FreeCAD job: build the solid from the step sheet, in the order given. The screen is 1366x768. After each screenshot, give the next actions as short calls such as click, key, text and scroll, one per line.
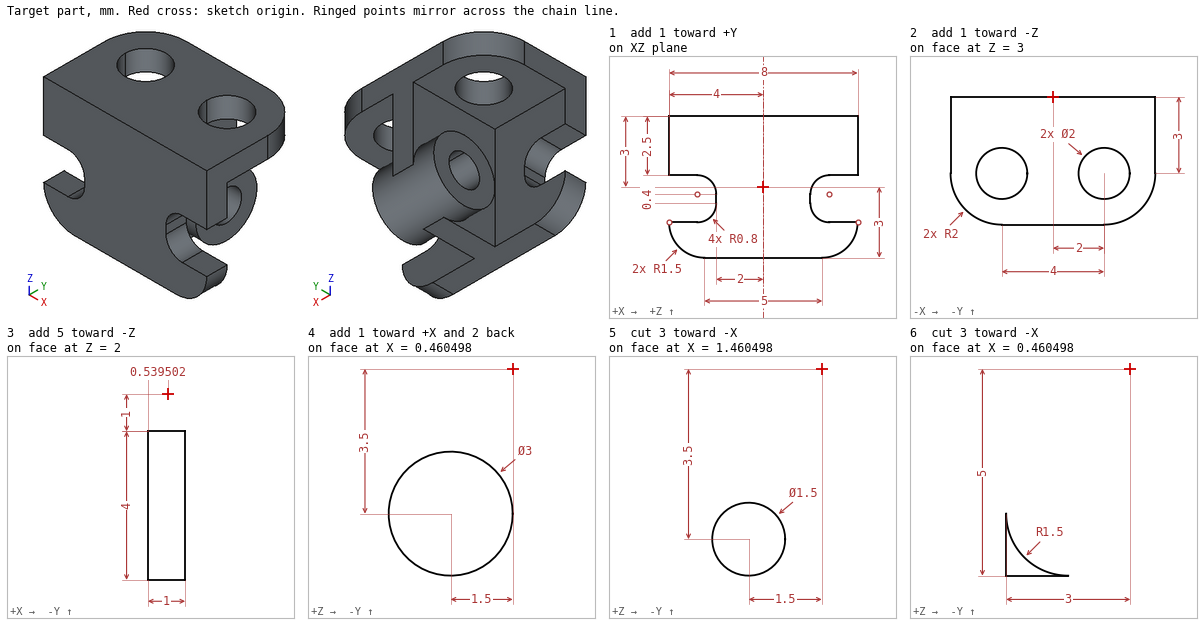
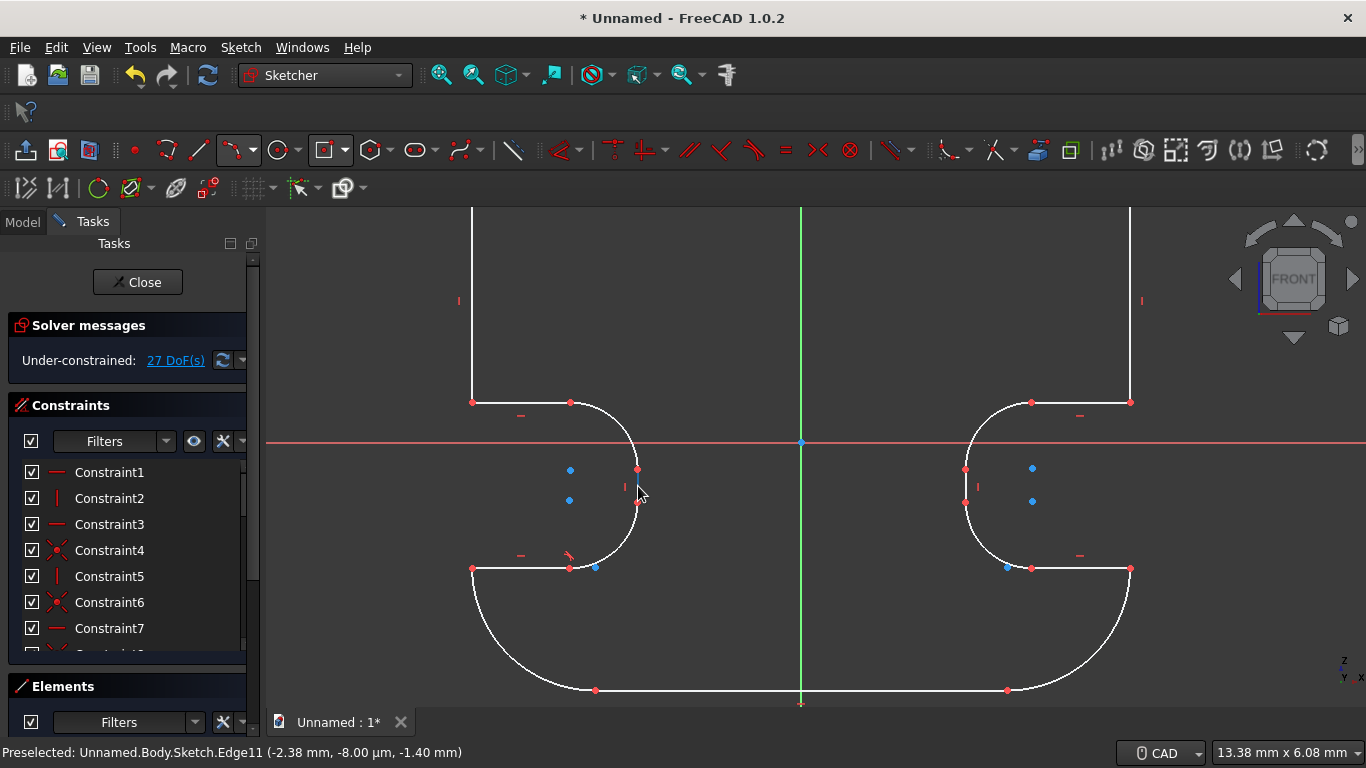
click(638, 486)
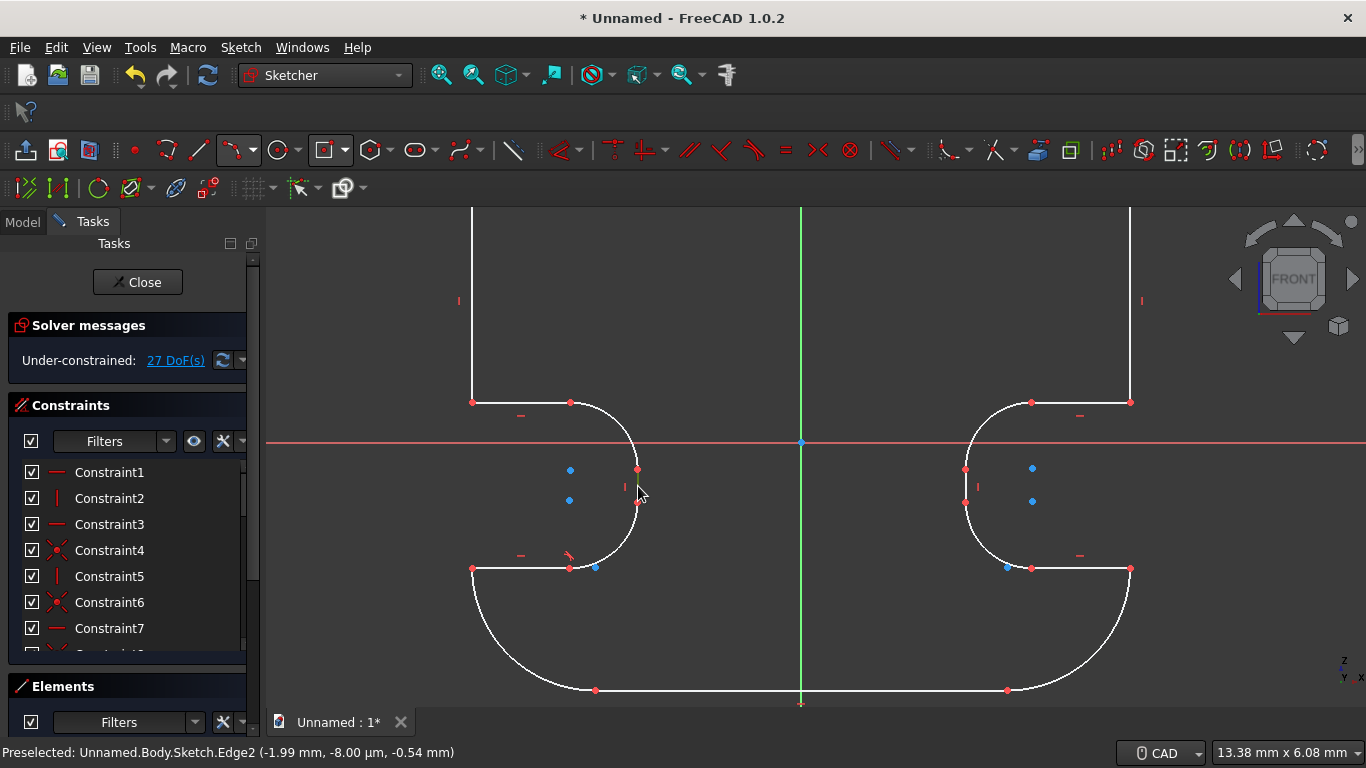
click(600, 561)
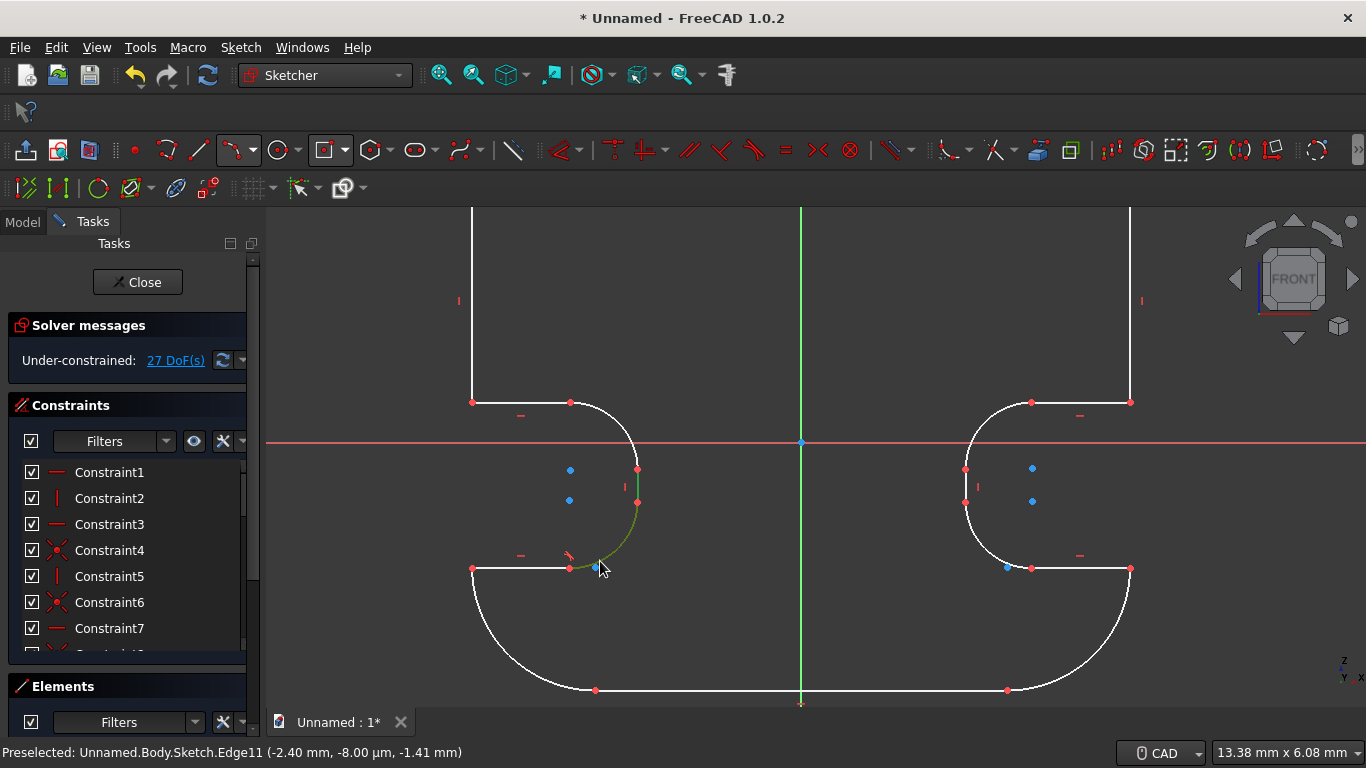
click(754, 150)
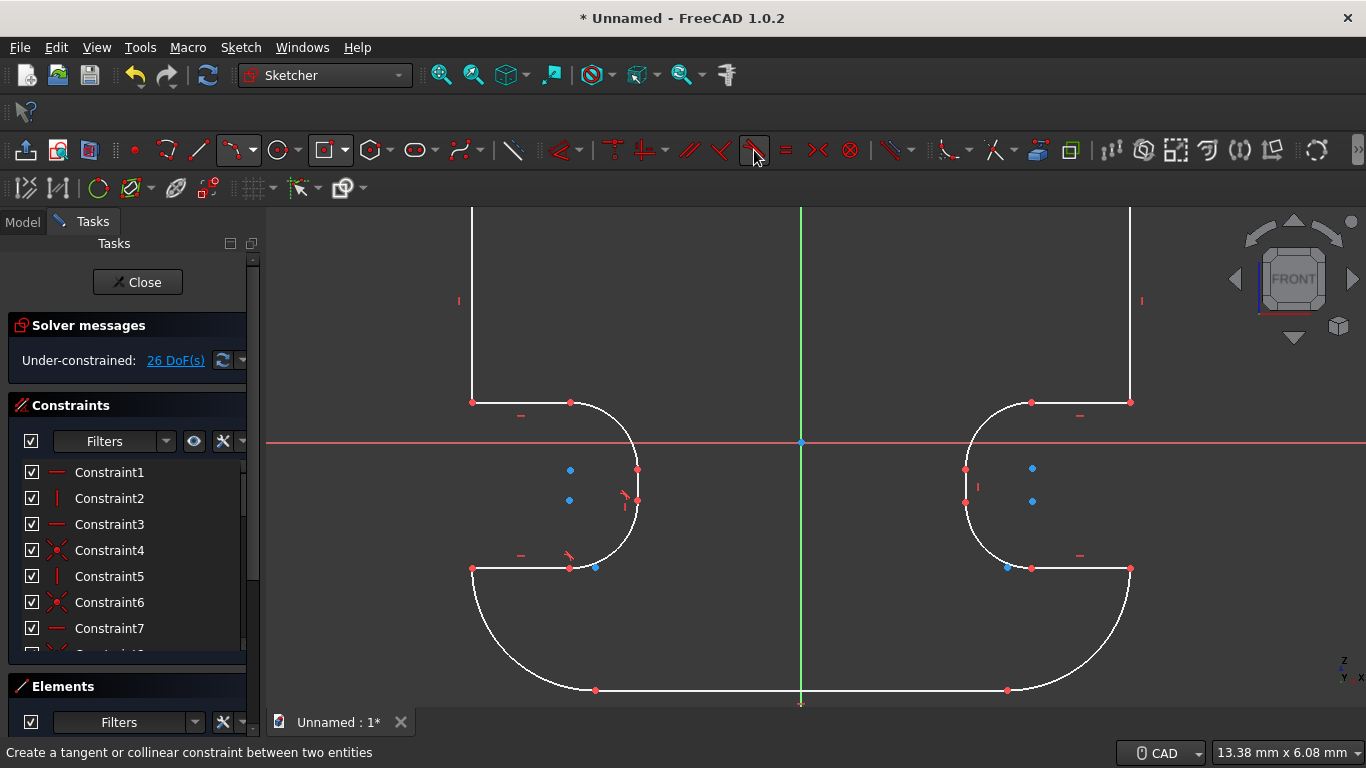
scroll(638, 491, up, 3)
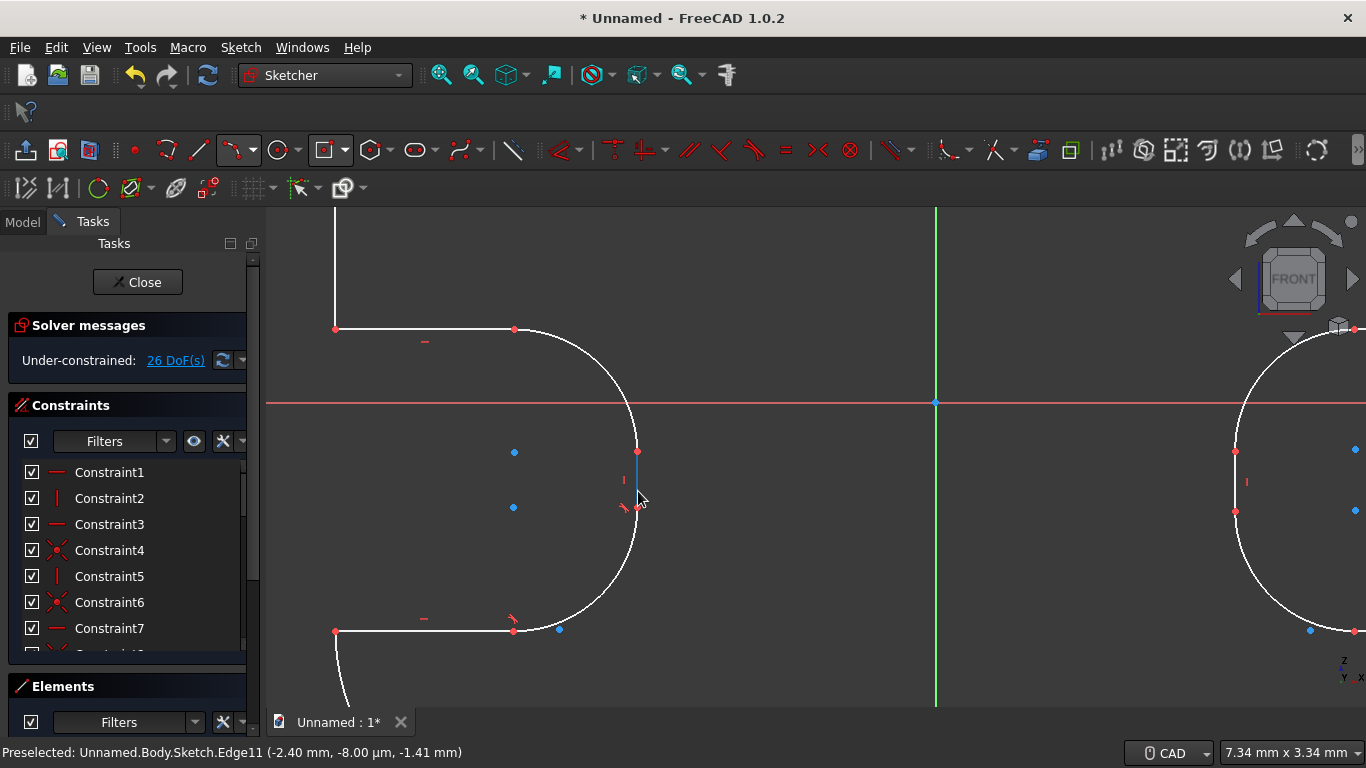
click(637, 491)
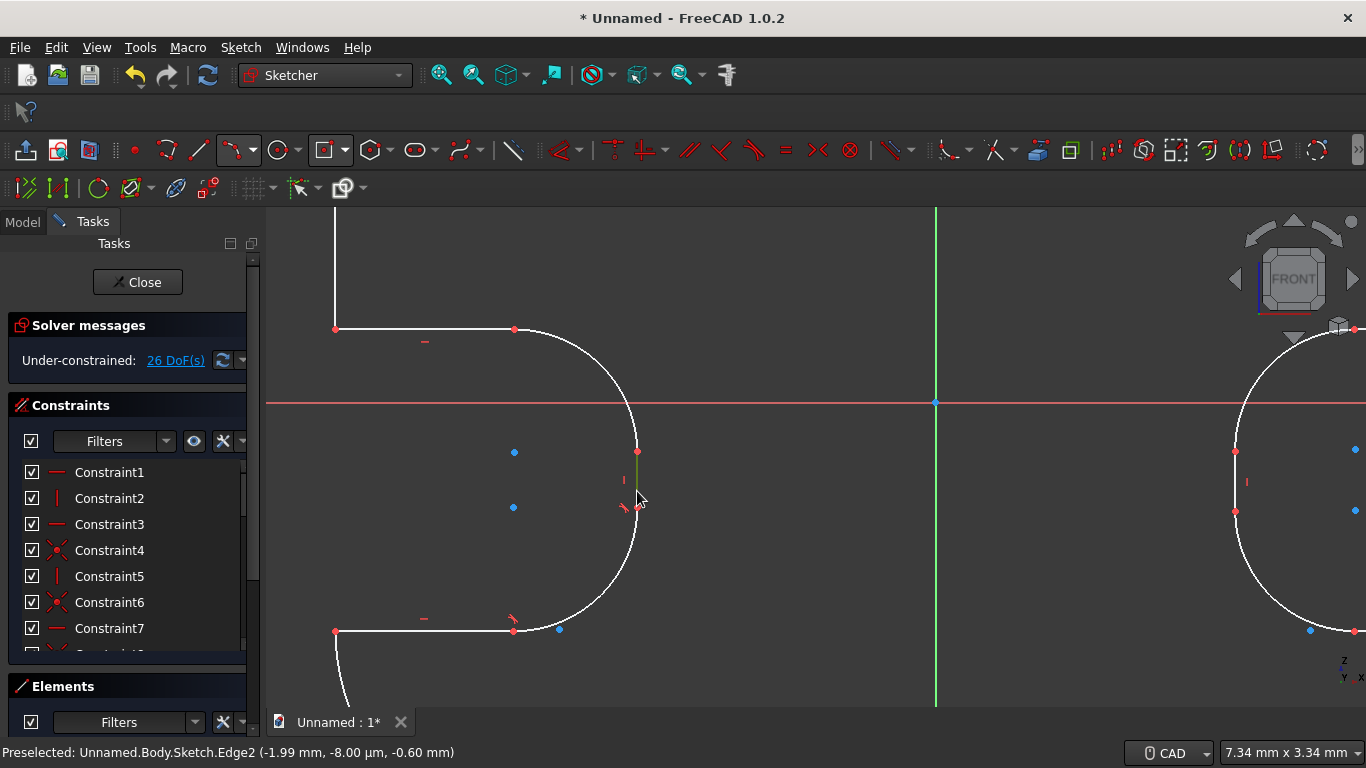
click(570, 343)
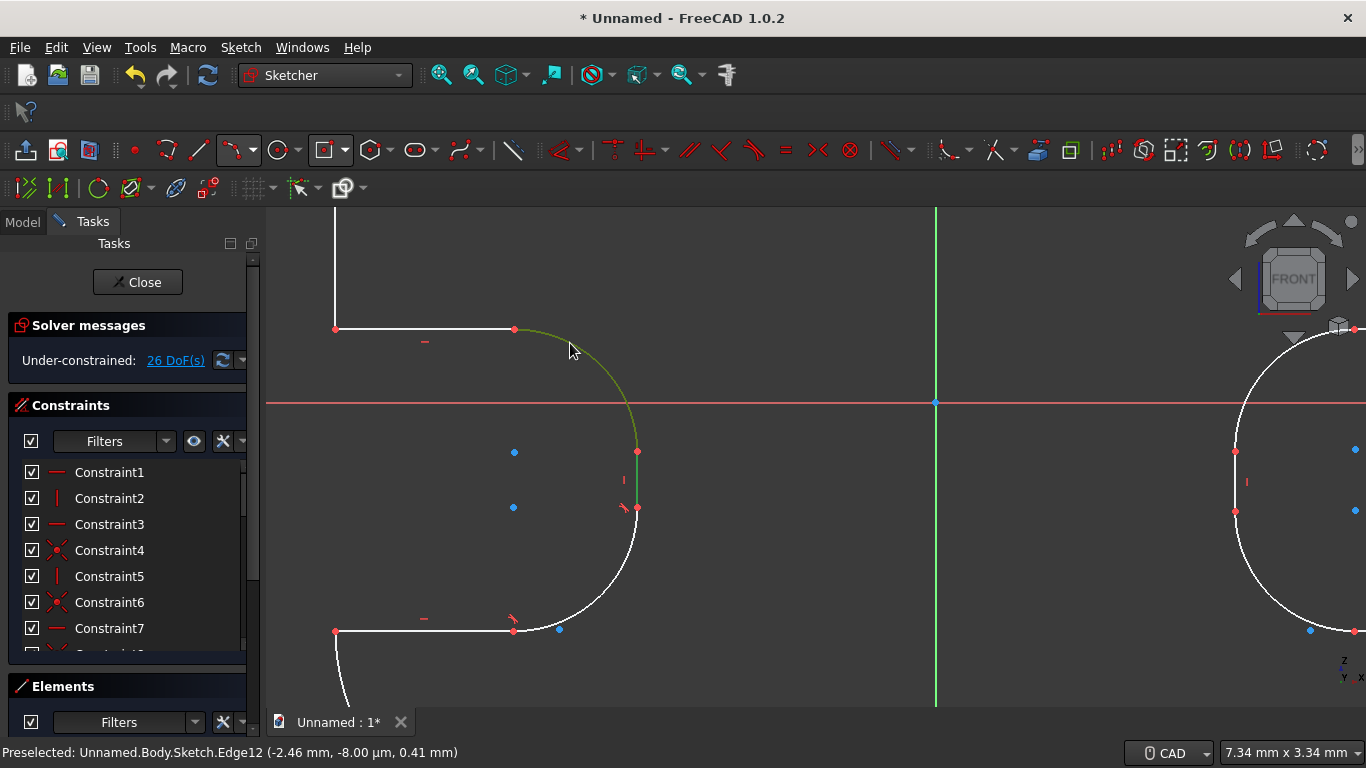
click(754, 150)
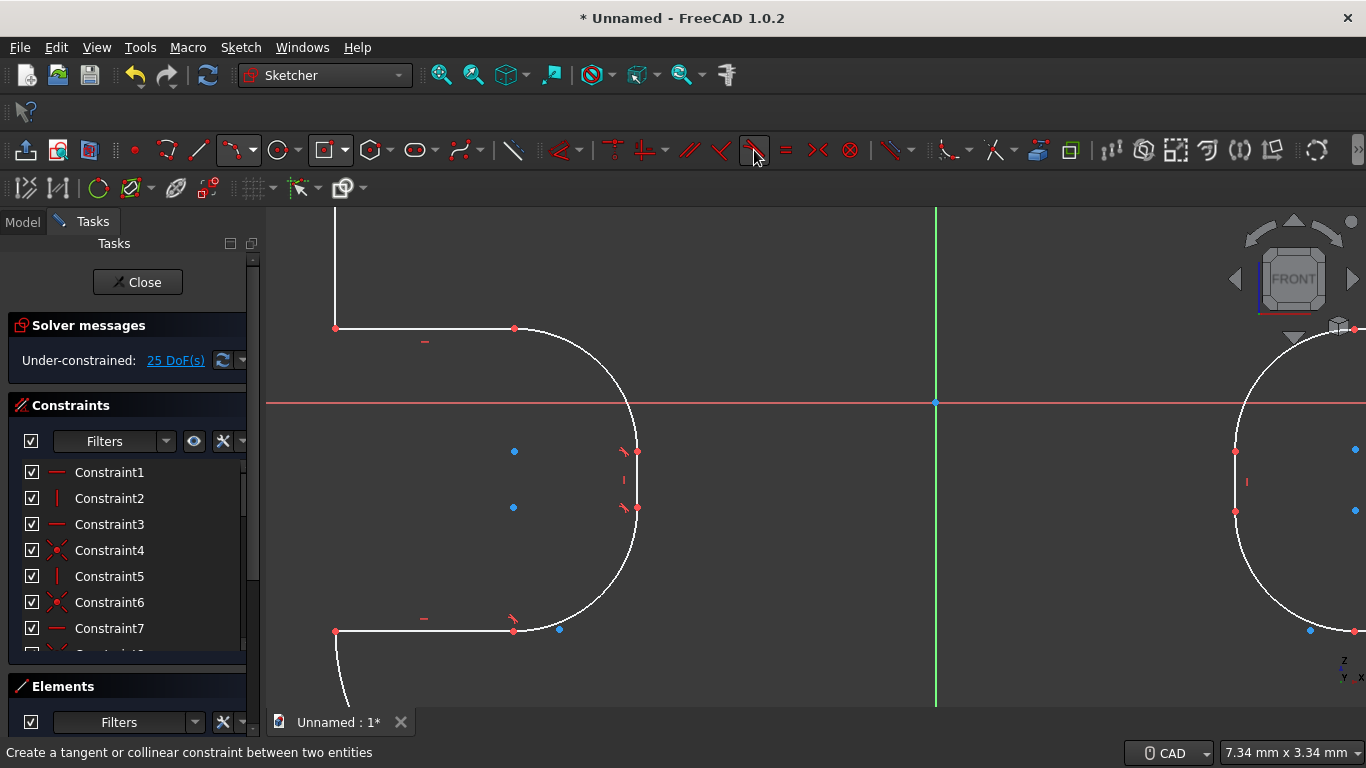
click(461, 329)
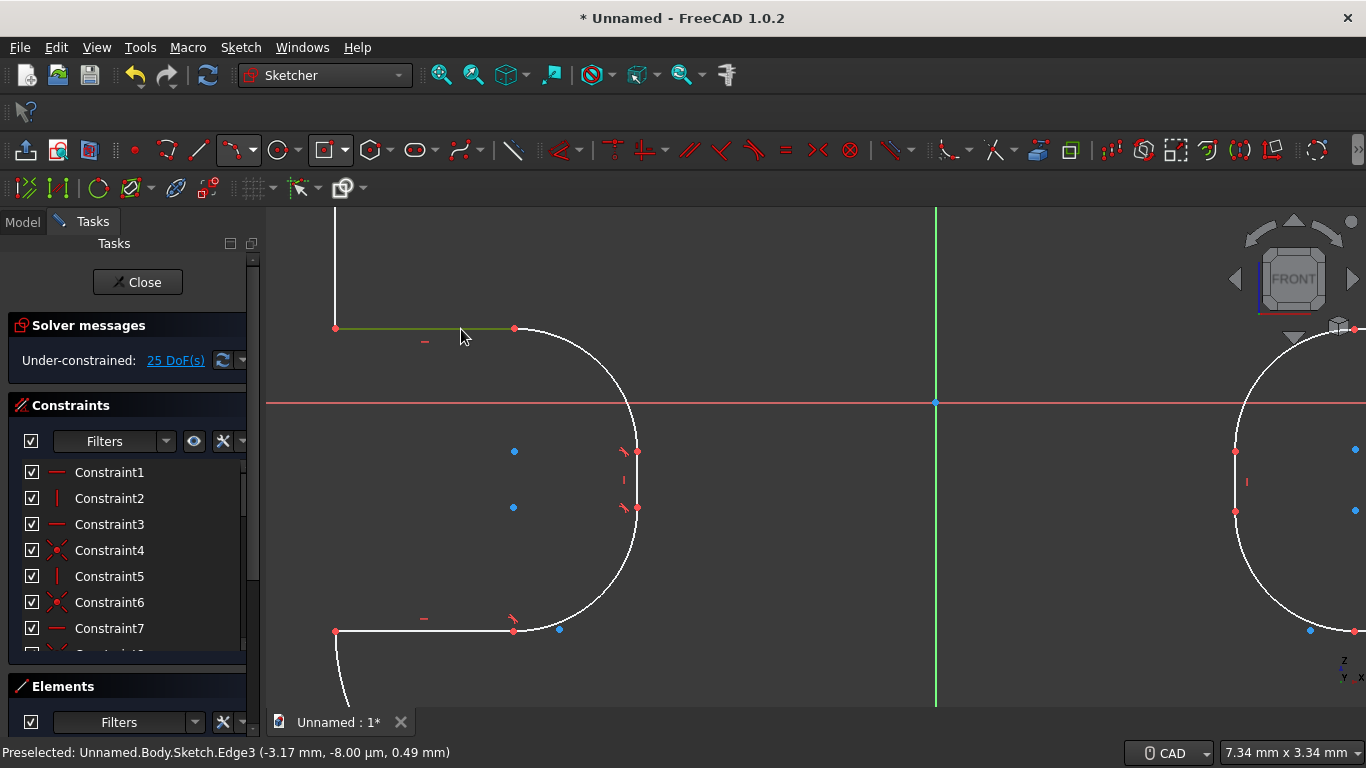
click(570, 342)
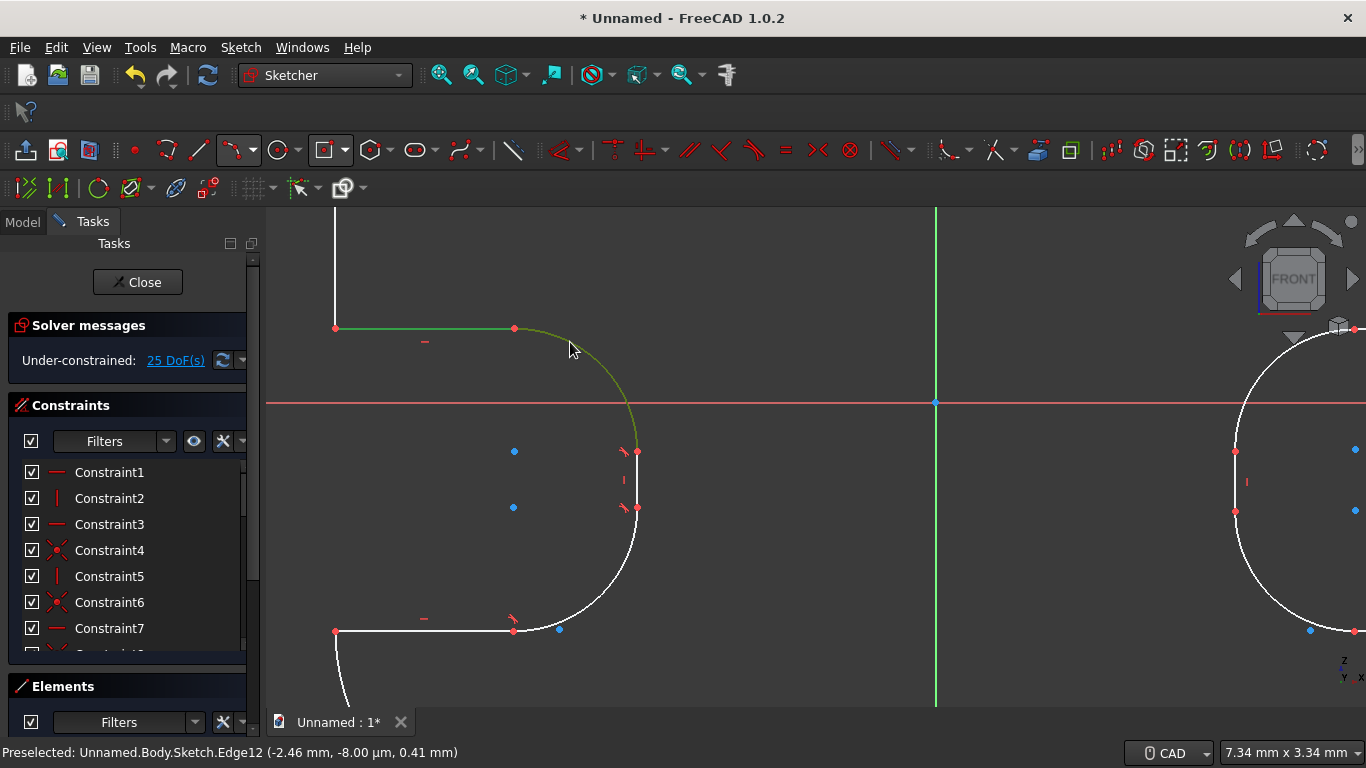
click(754, 150)